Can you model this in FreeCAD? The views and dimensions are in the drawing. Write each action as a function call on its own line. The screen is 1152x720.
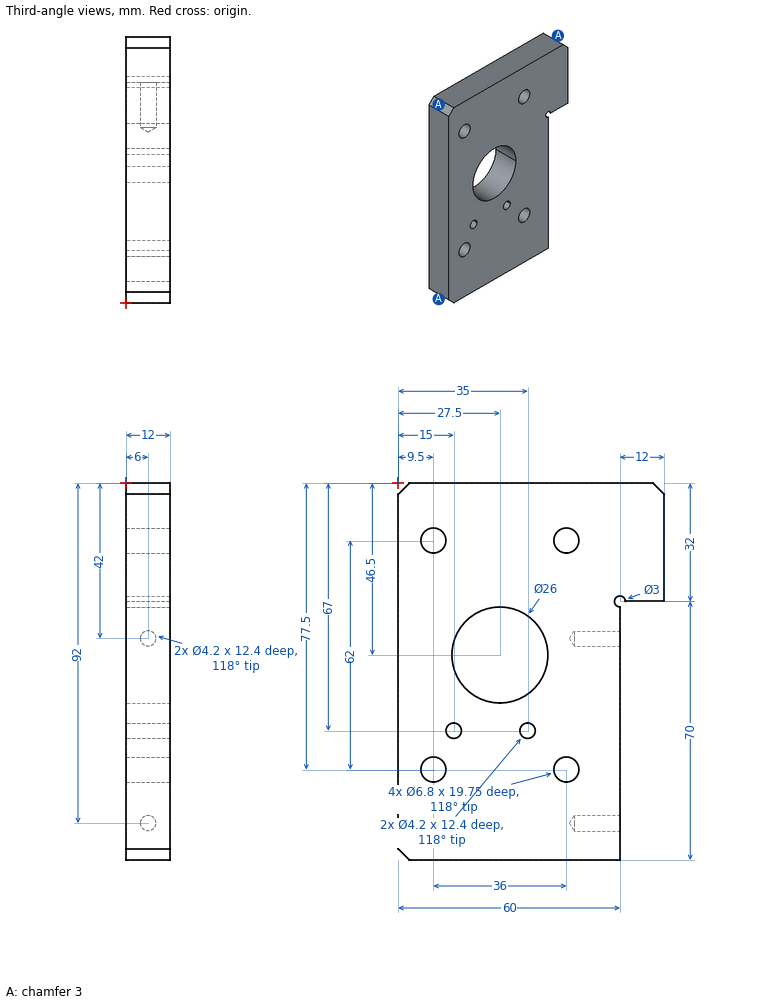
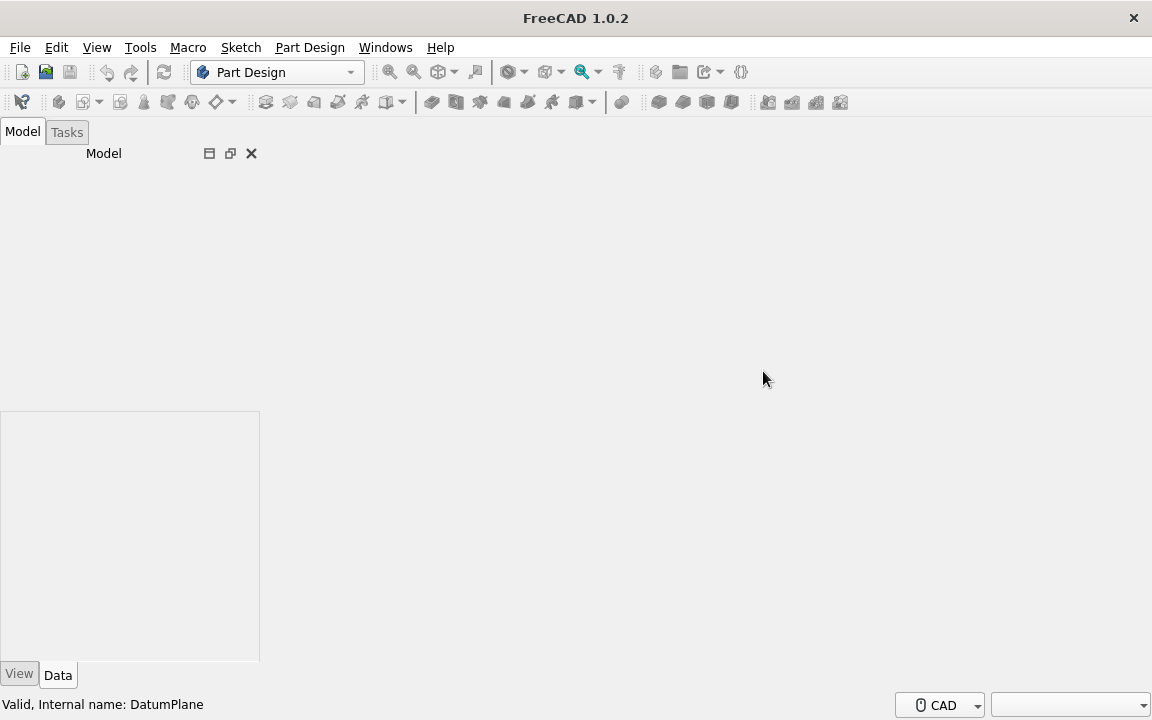
click(22, 72)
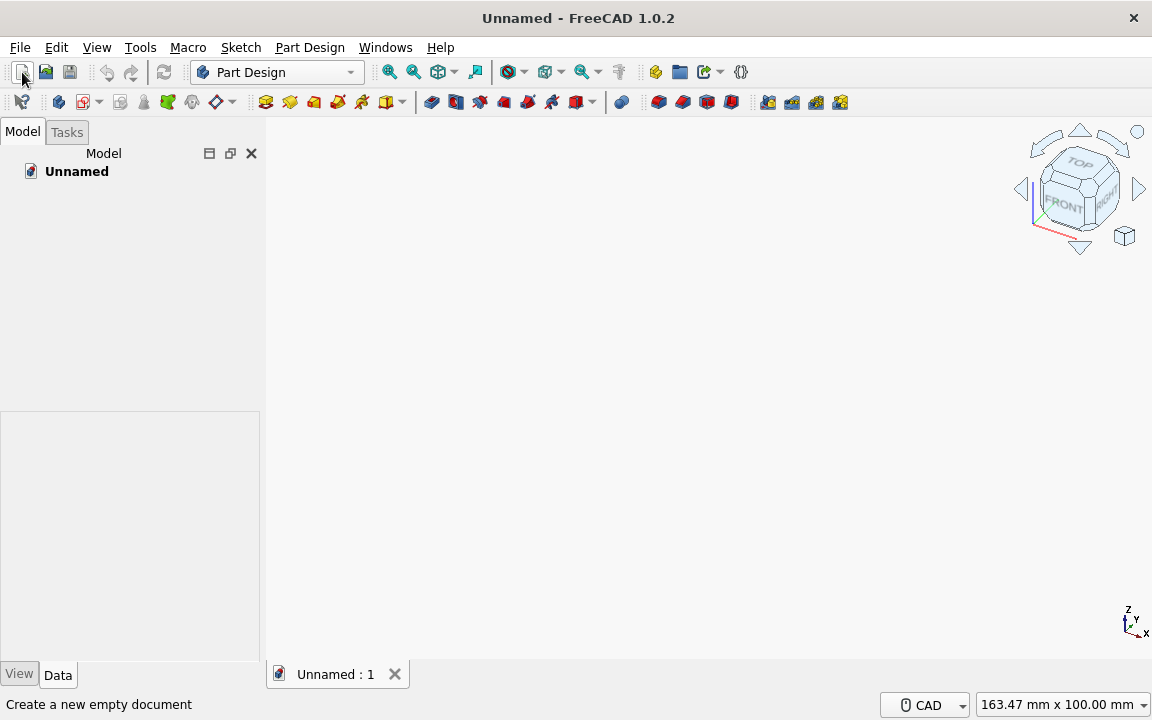
click(84, 102)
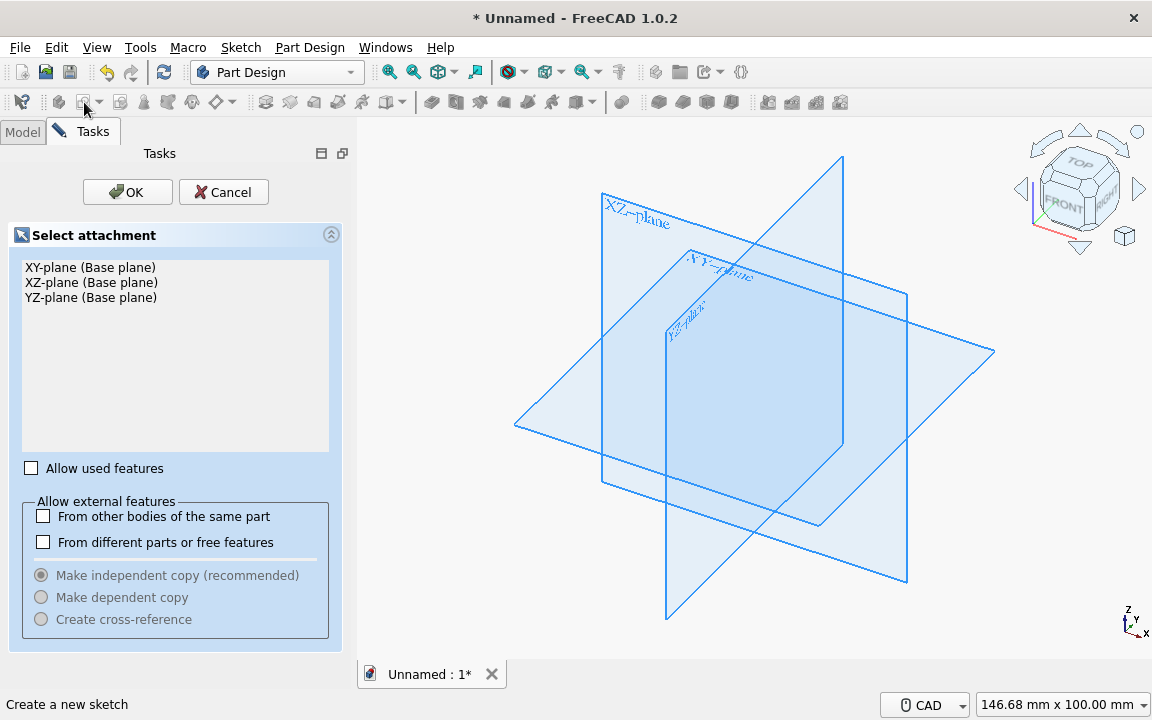
click(82, 298)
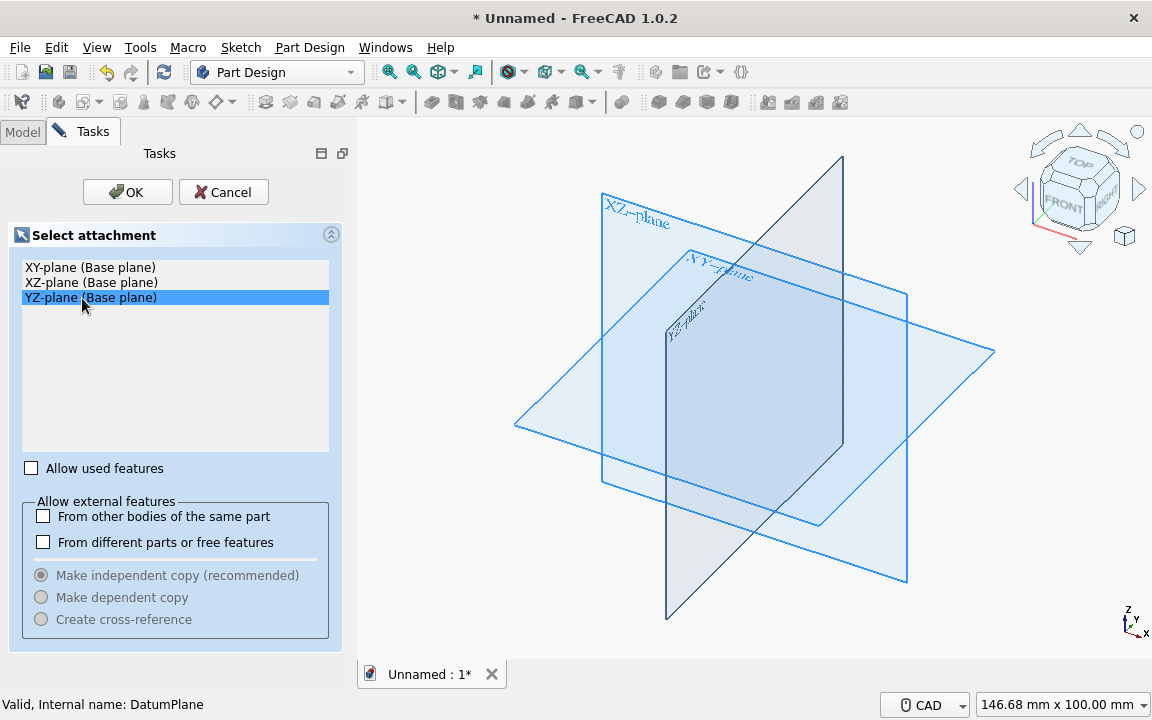
click(128, 192)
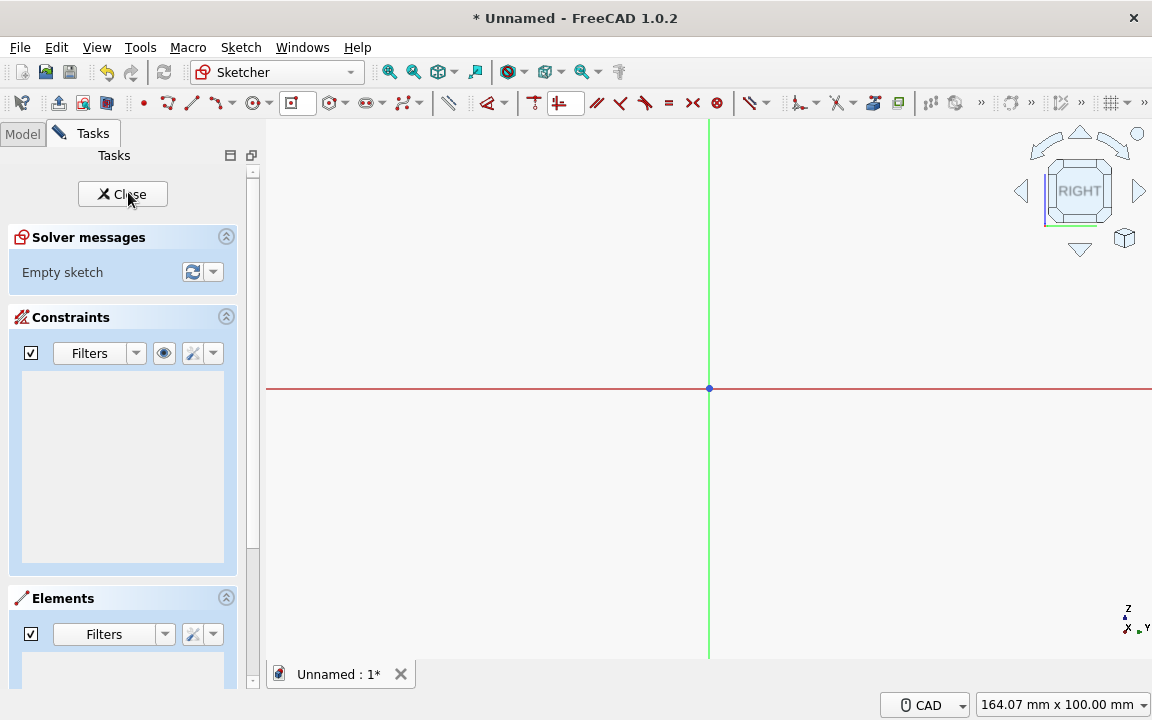
scroll(321, 147, down, 3)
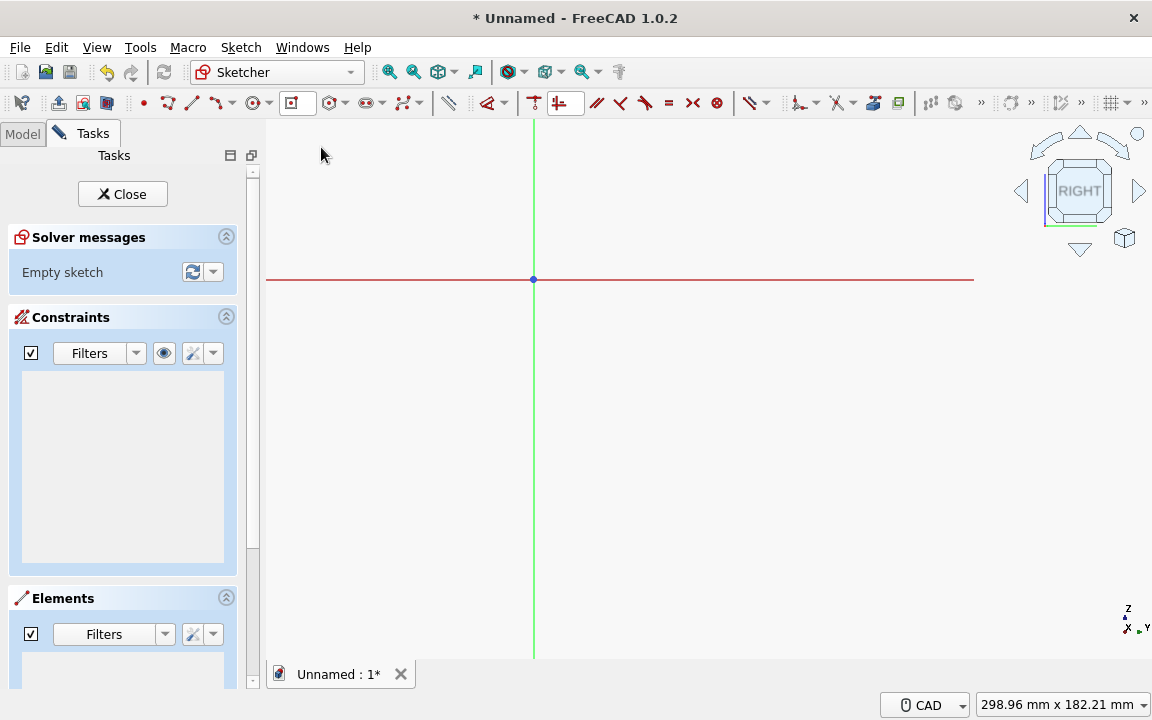
click(168, 104)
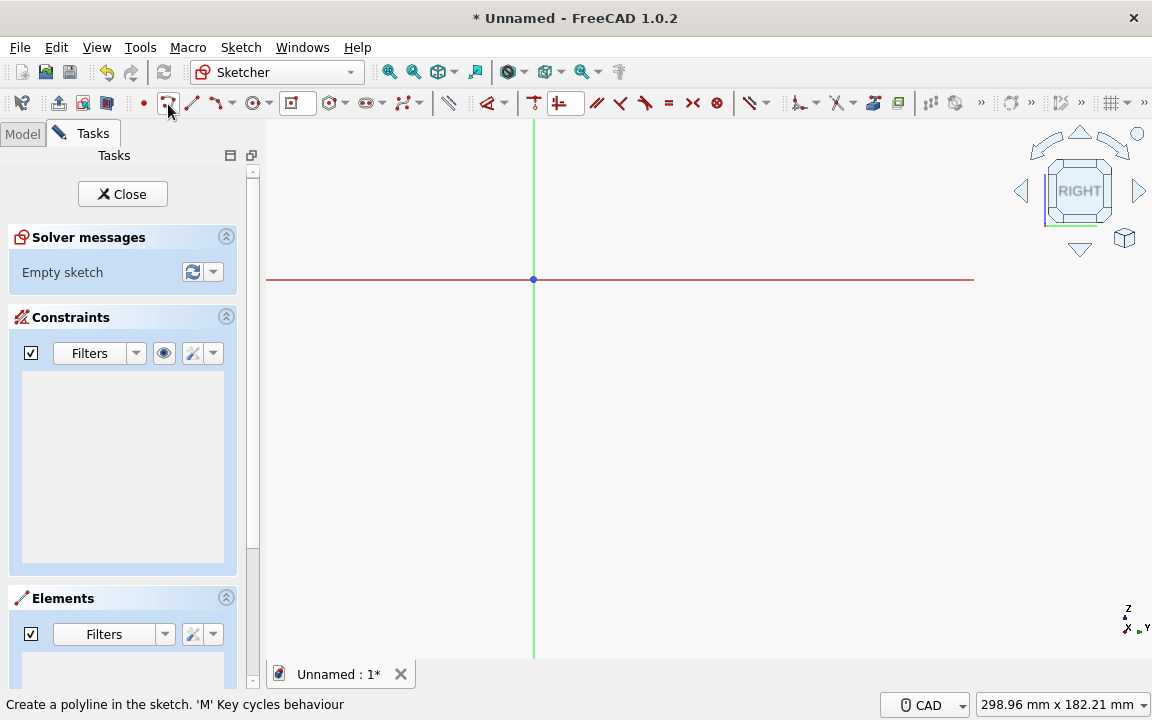
click(534, 280)
click(543, 582)
click(712, 582)
click(712, 375)
click(747, 375)
click(747, 289)
click(534, 280)
key(Escape)
key(Escape)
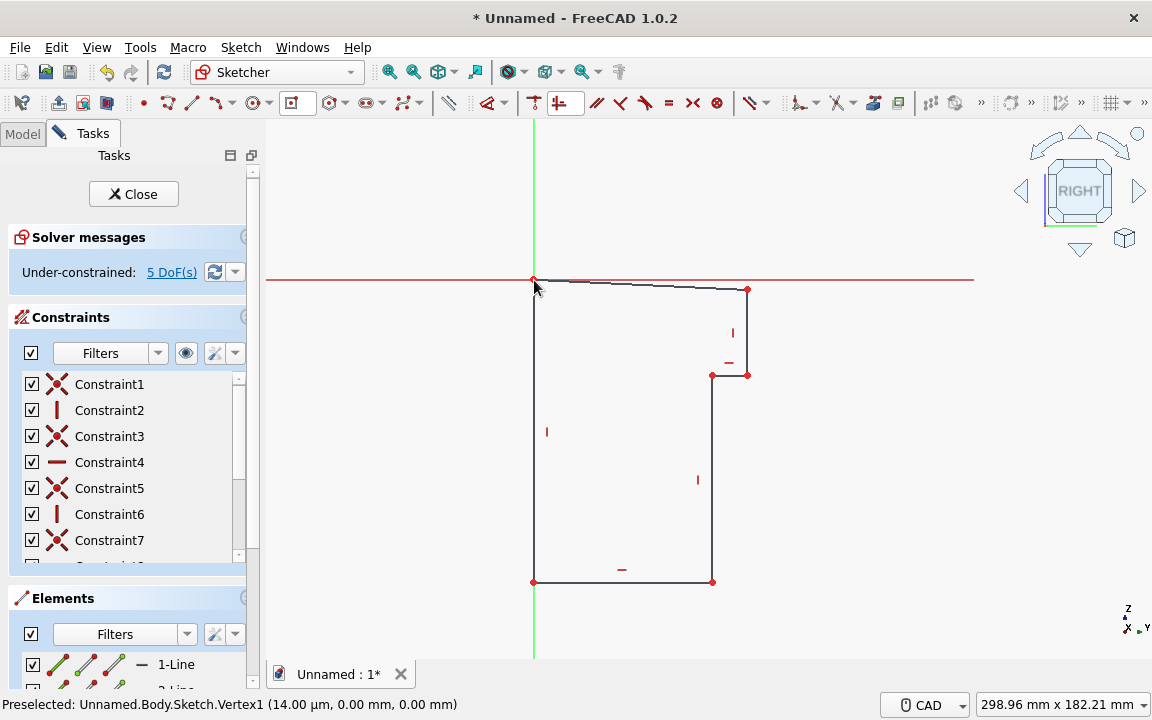
click(598, 283)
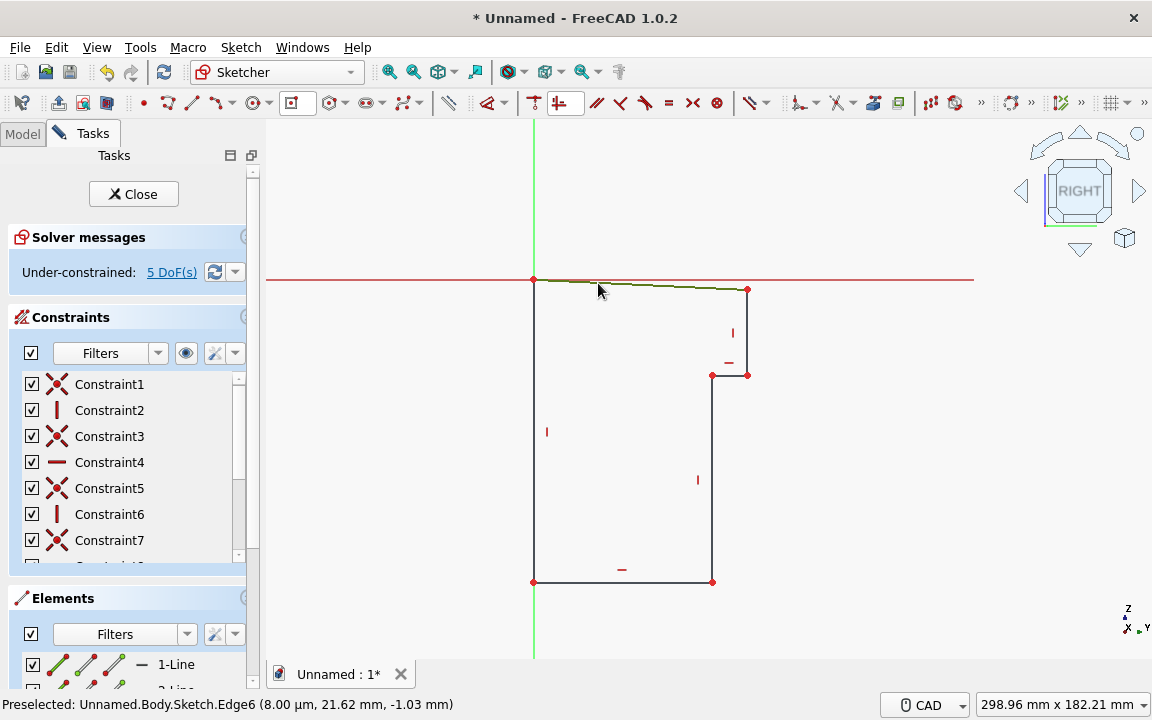
click(578, 104)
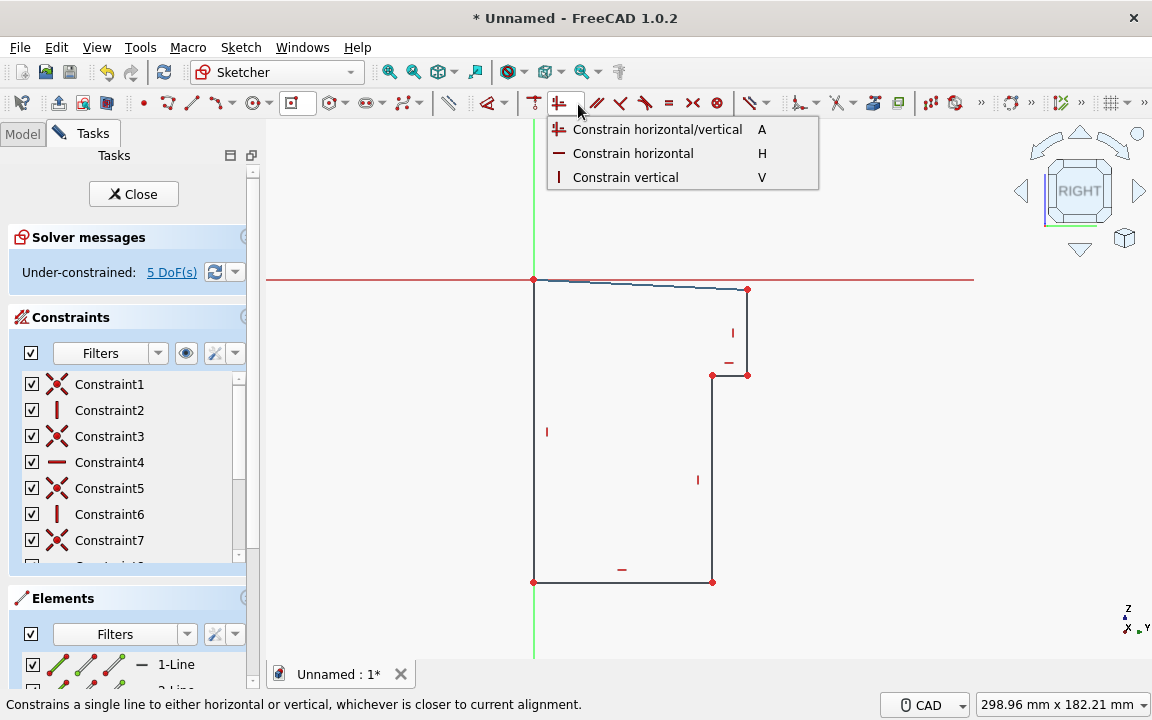
click(683, 153)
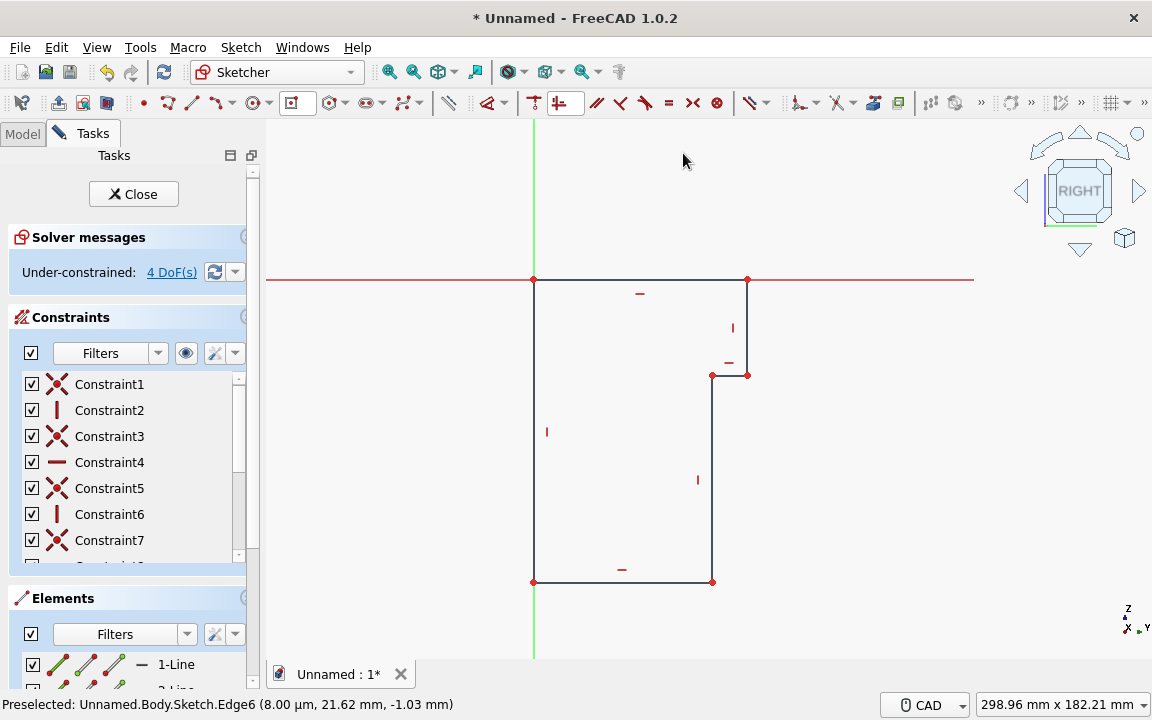
click(587, 583)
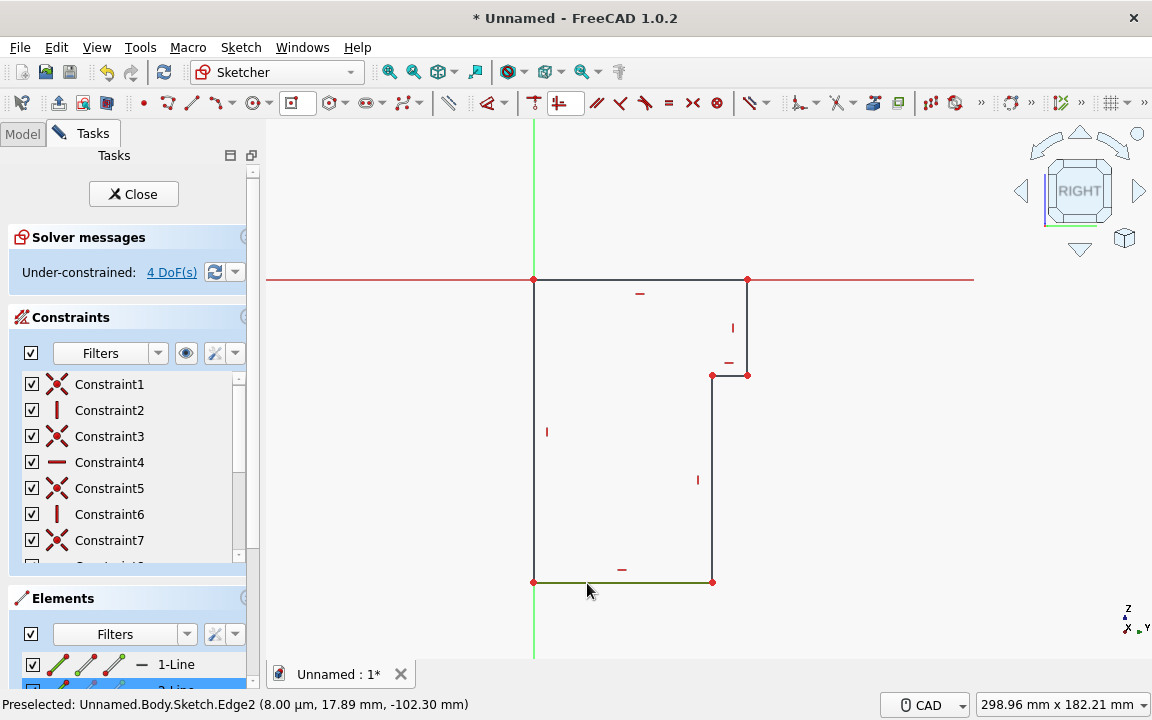
key(l)